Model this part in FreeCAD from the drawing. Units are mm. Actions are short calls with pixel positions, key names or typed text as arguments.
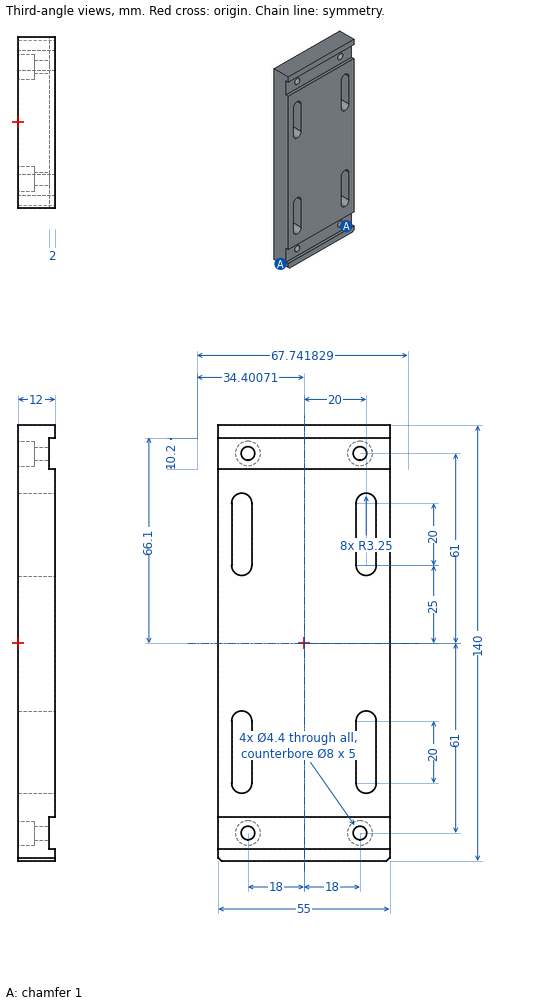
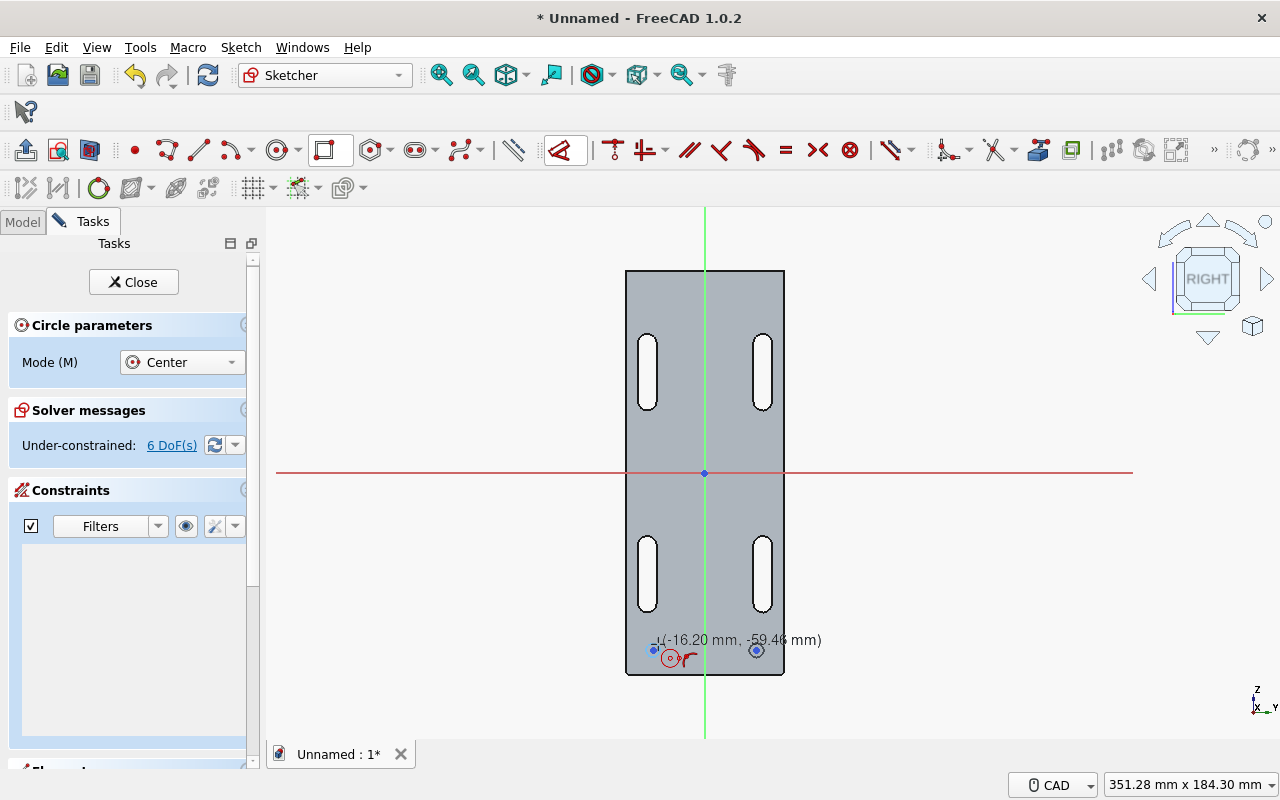
scroll(757, 297, up, 7)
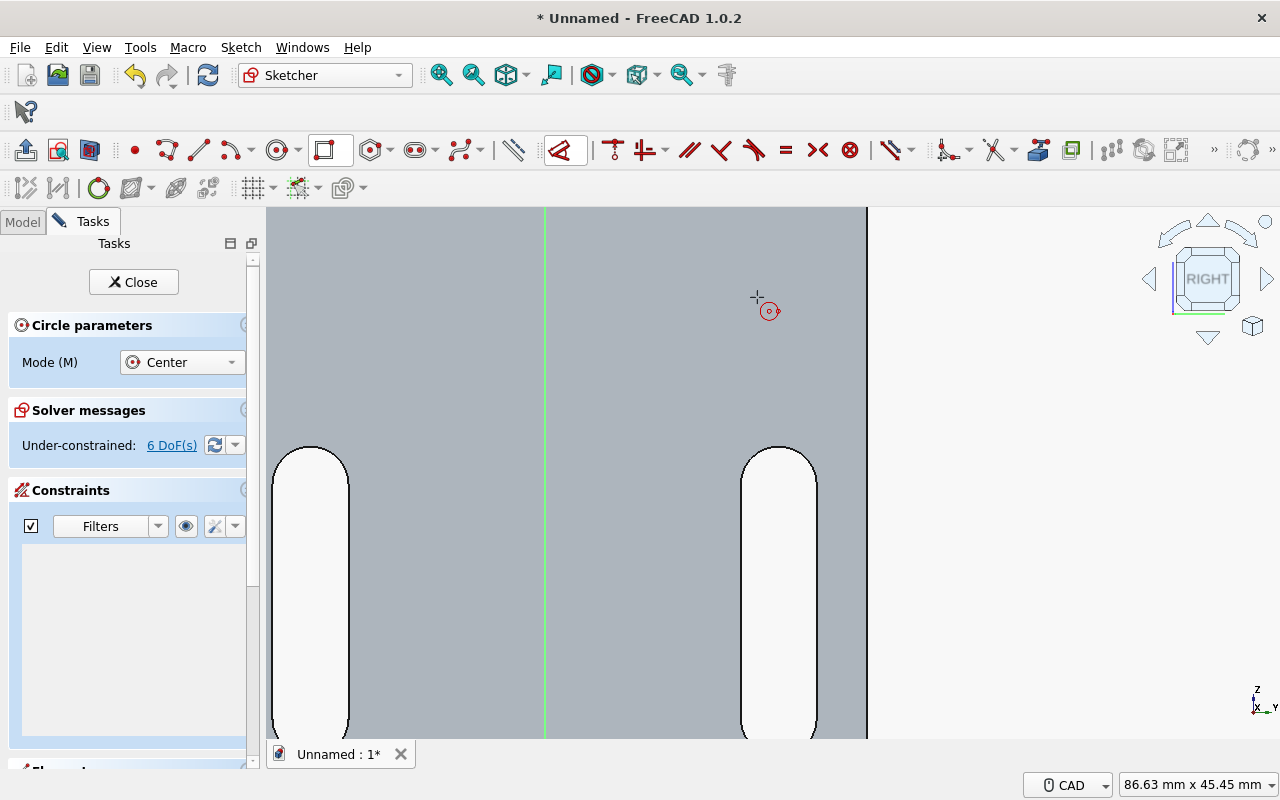
scroll(757, 297, down, 7)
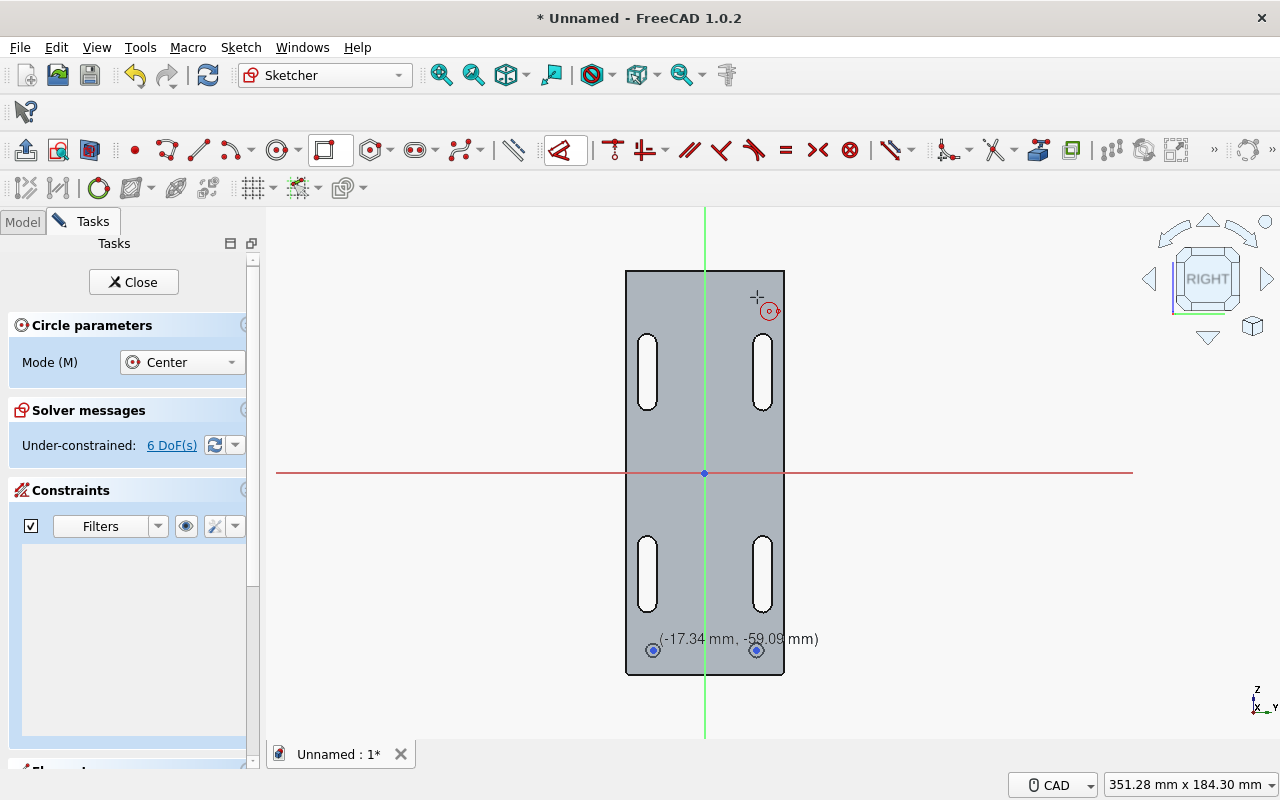
click(757, 297)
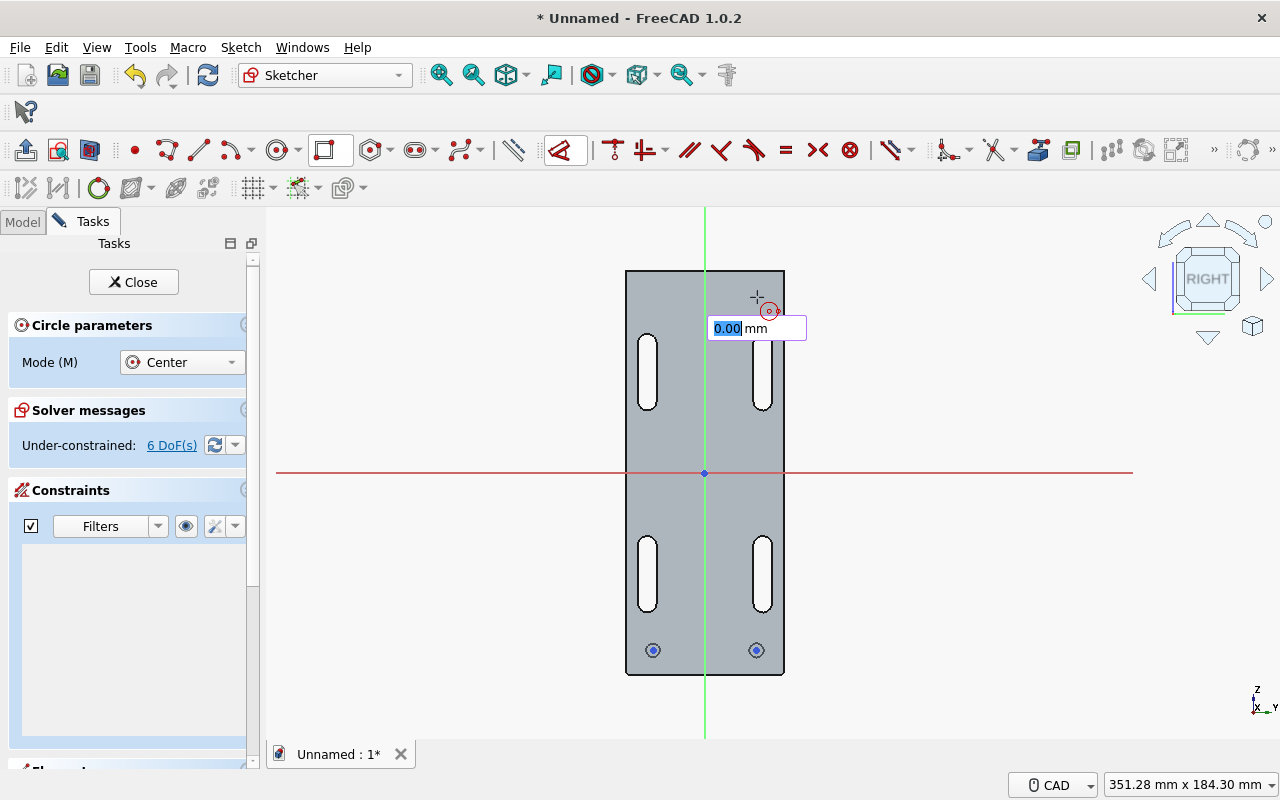
scroll(761, 293, up, 5)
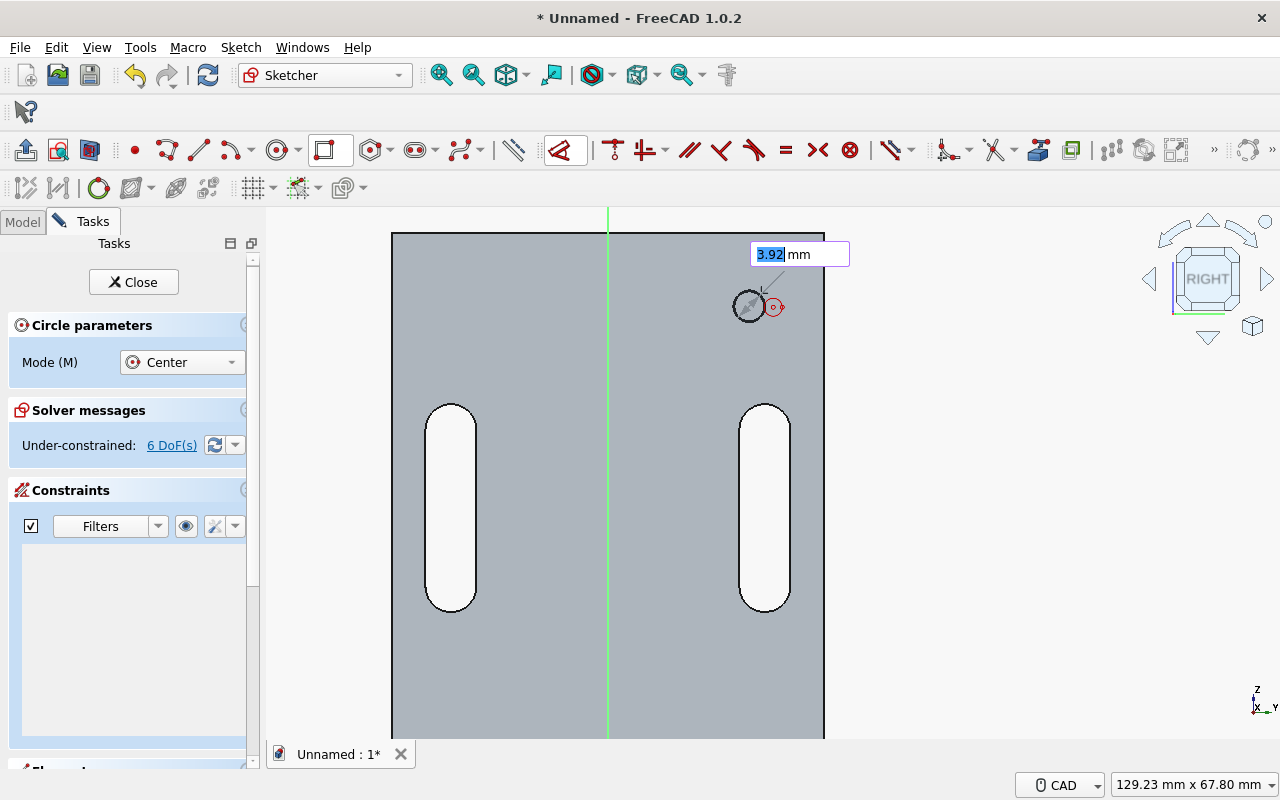
click(761, 292)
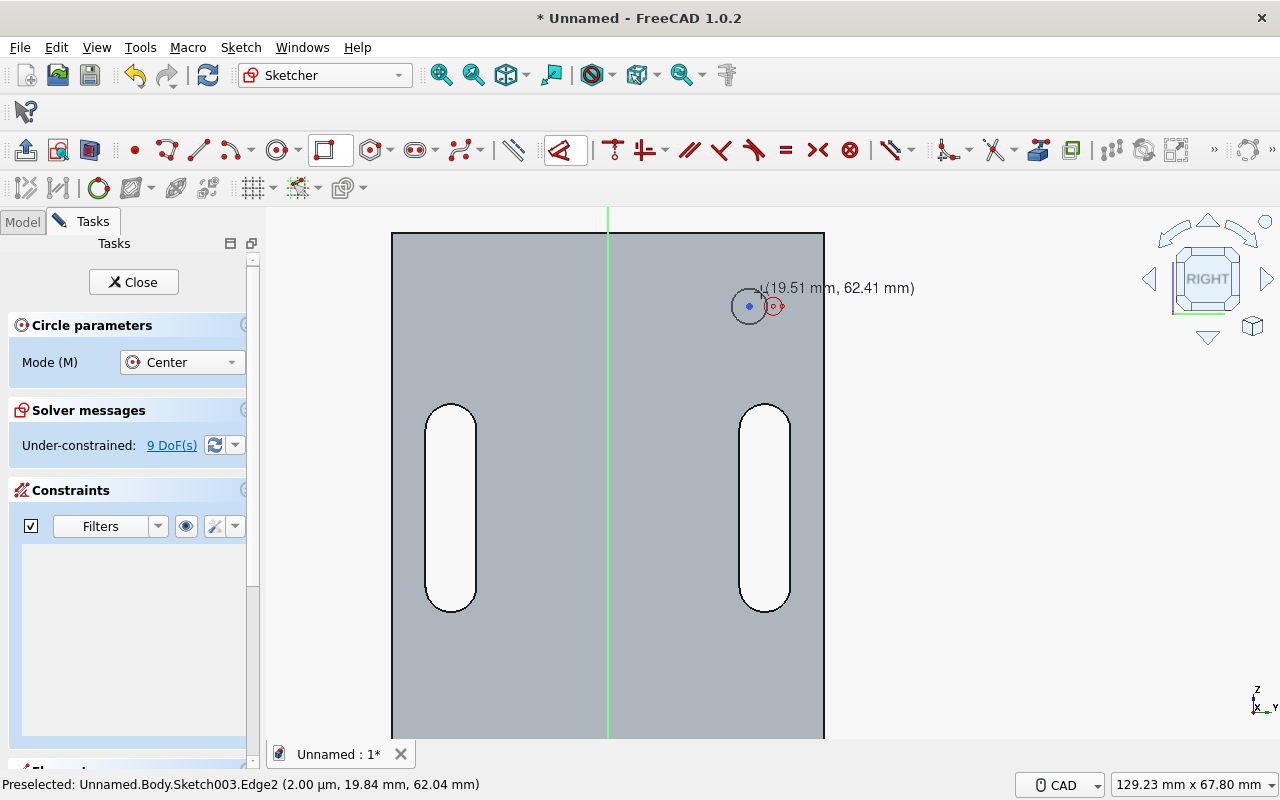
scroll(467, 304, up, 2)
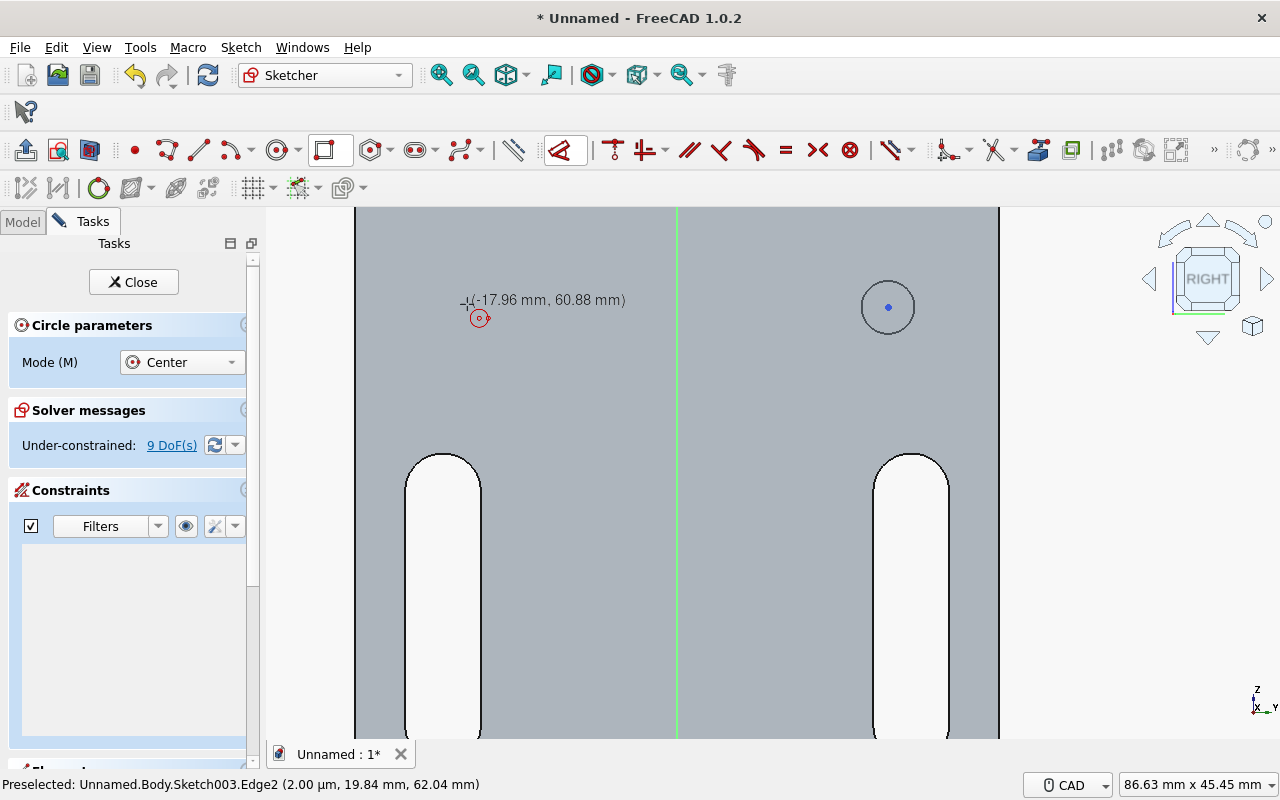
scroll(713, 295, down, 7)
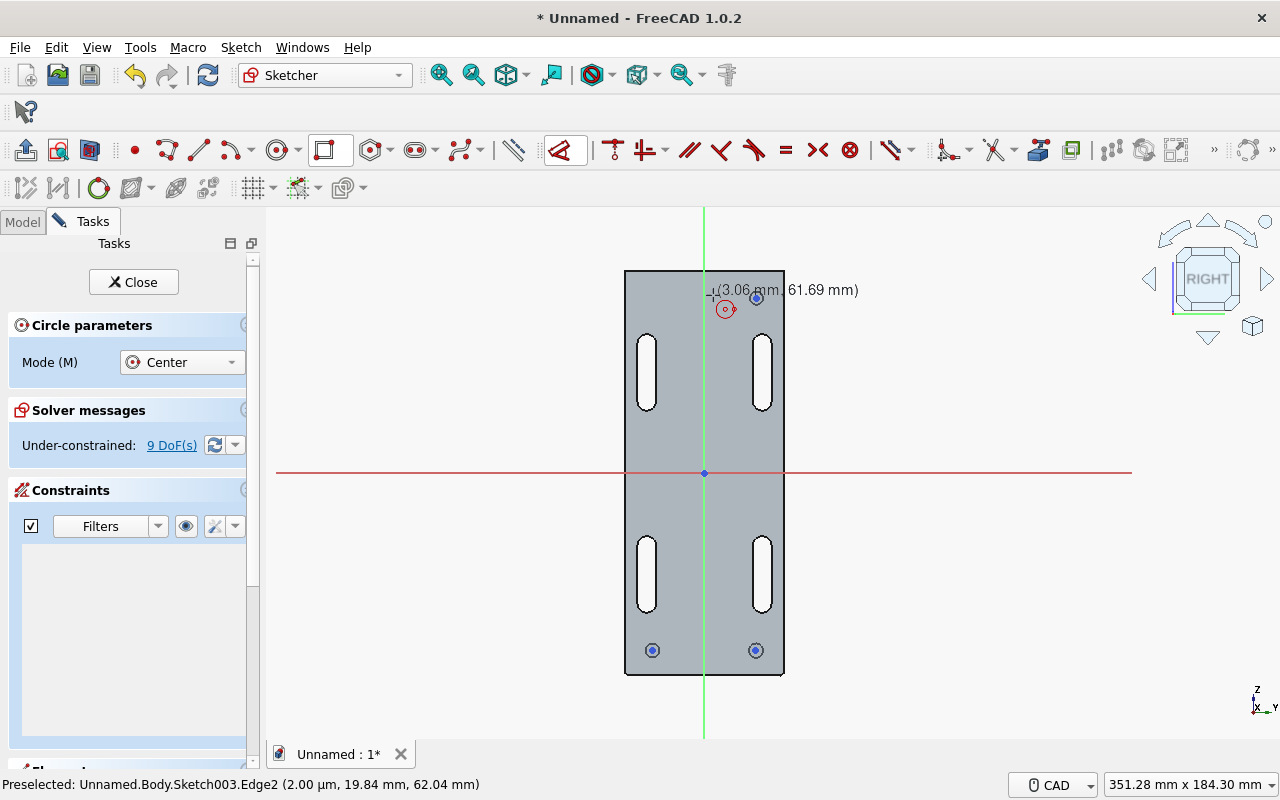
click(653, 297)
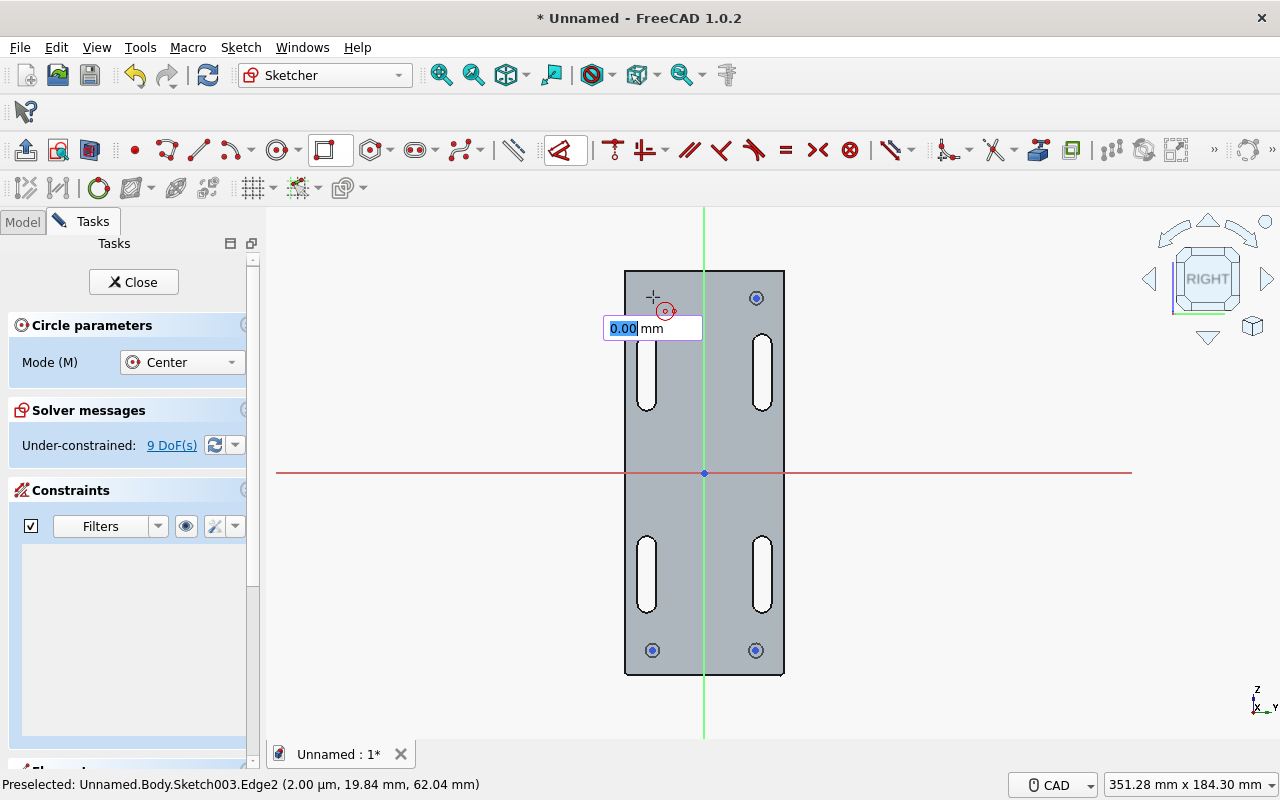
scroll(657, 293, up, 5)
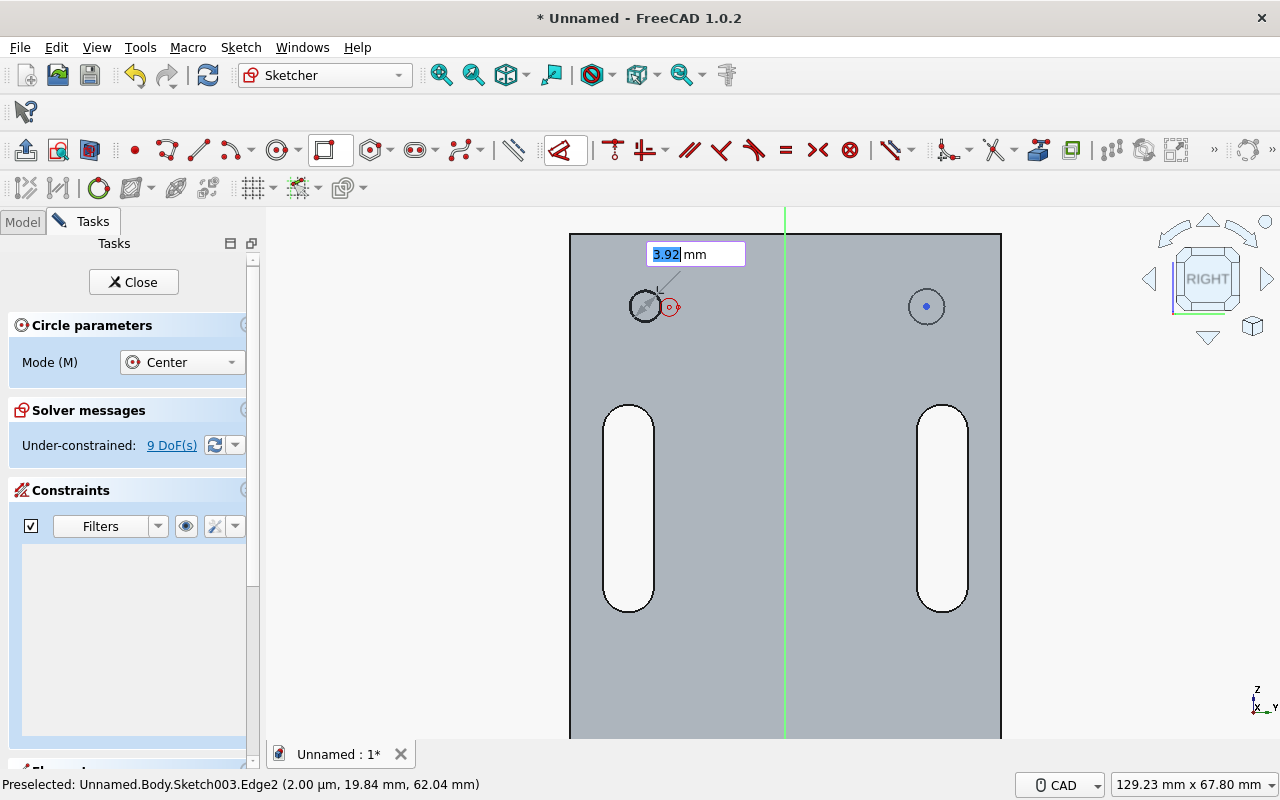
click(656, 292)
key(Escape)